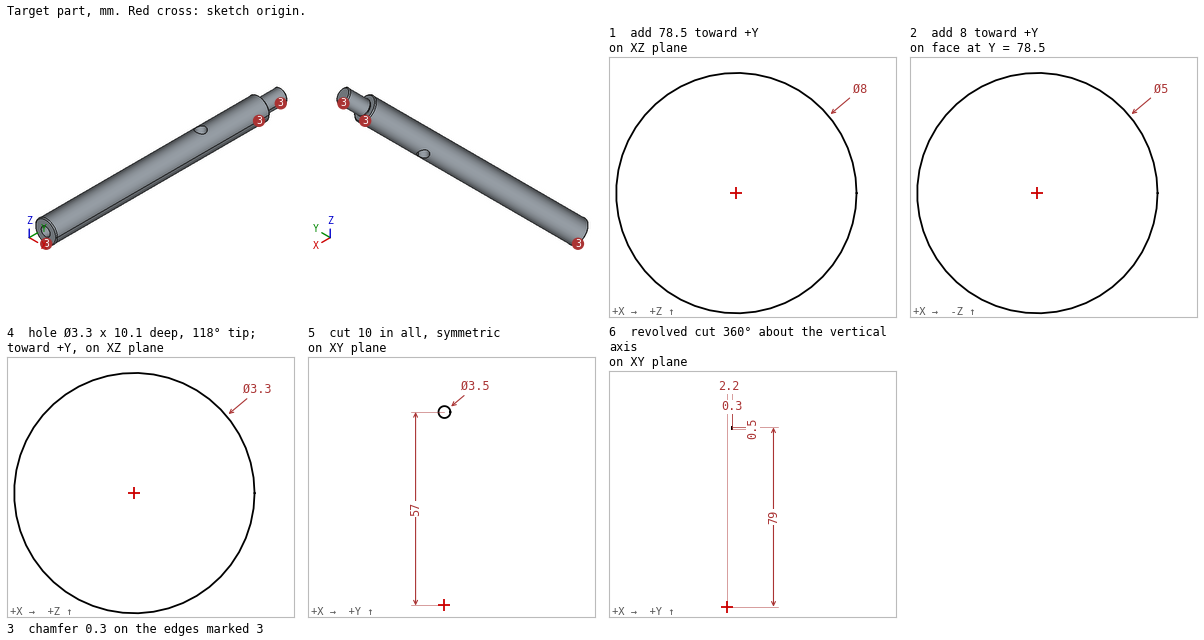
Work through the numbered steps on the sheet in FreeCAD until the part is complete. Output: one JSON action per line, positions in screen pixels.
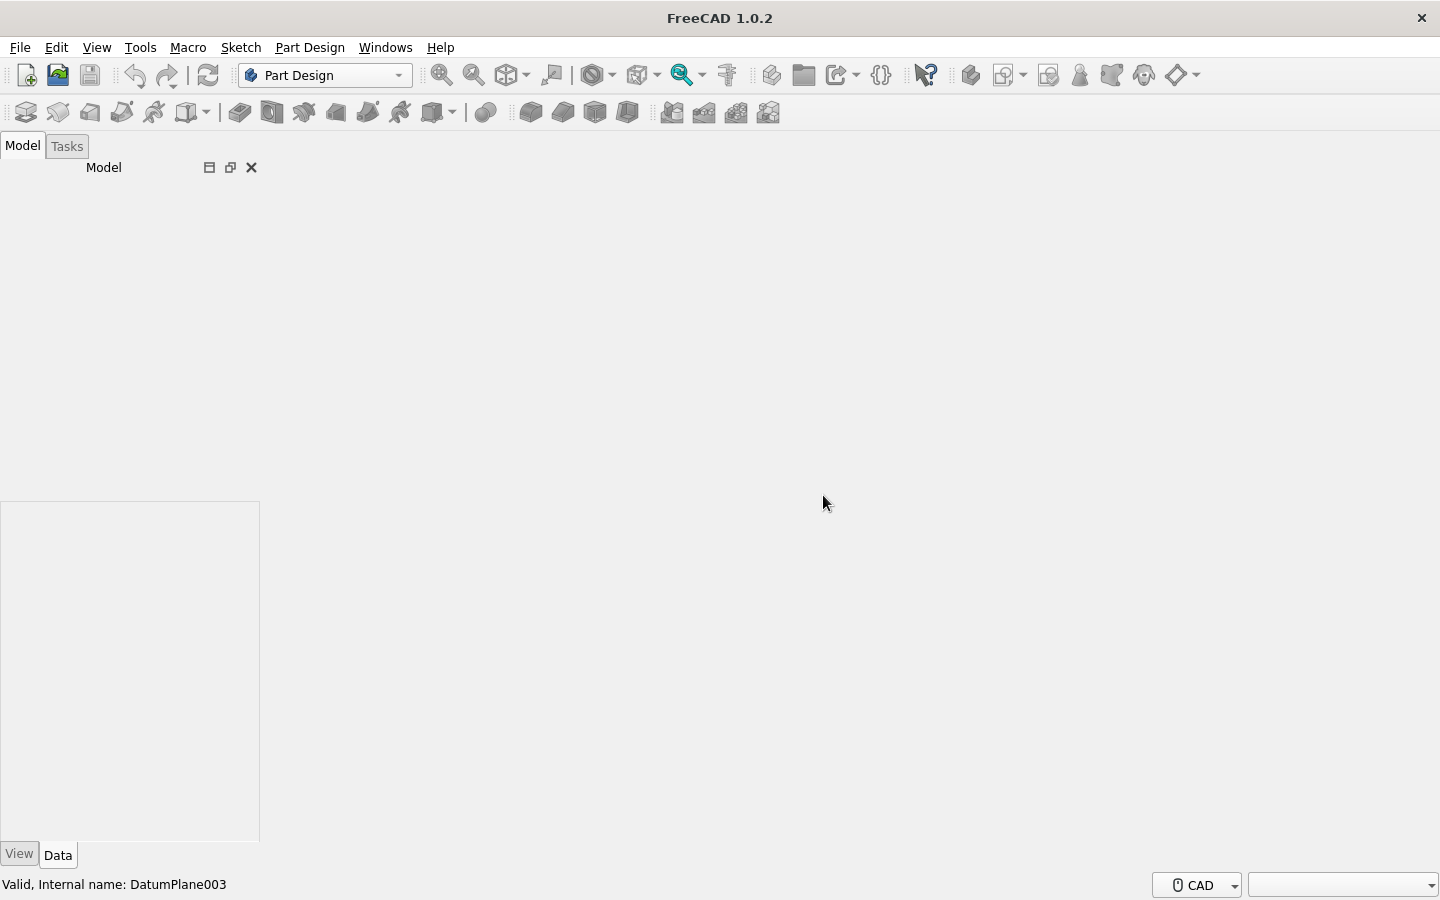
{"action": "left_click", "coordinate": [26, 76]}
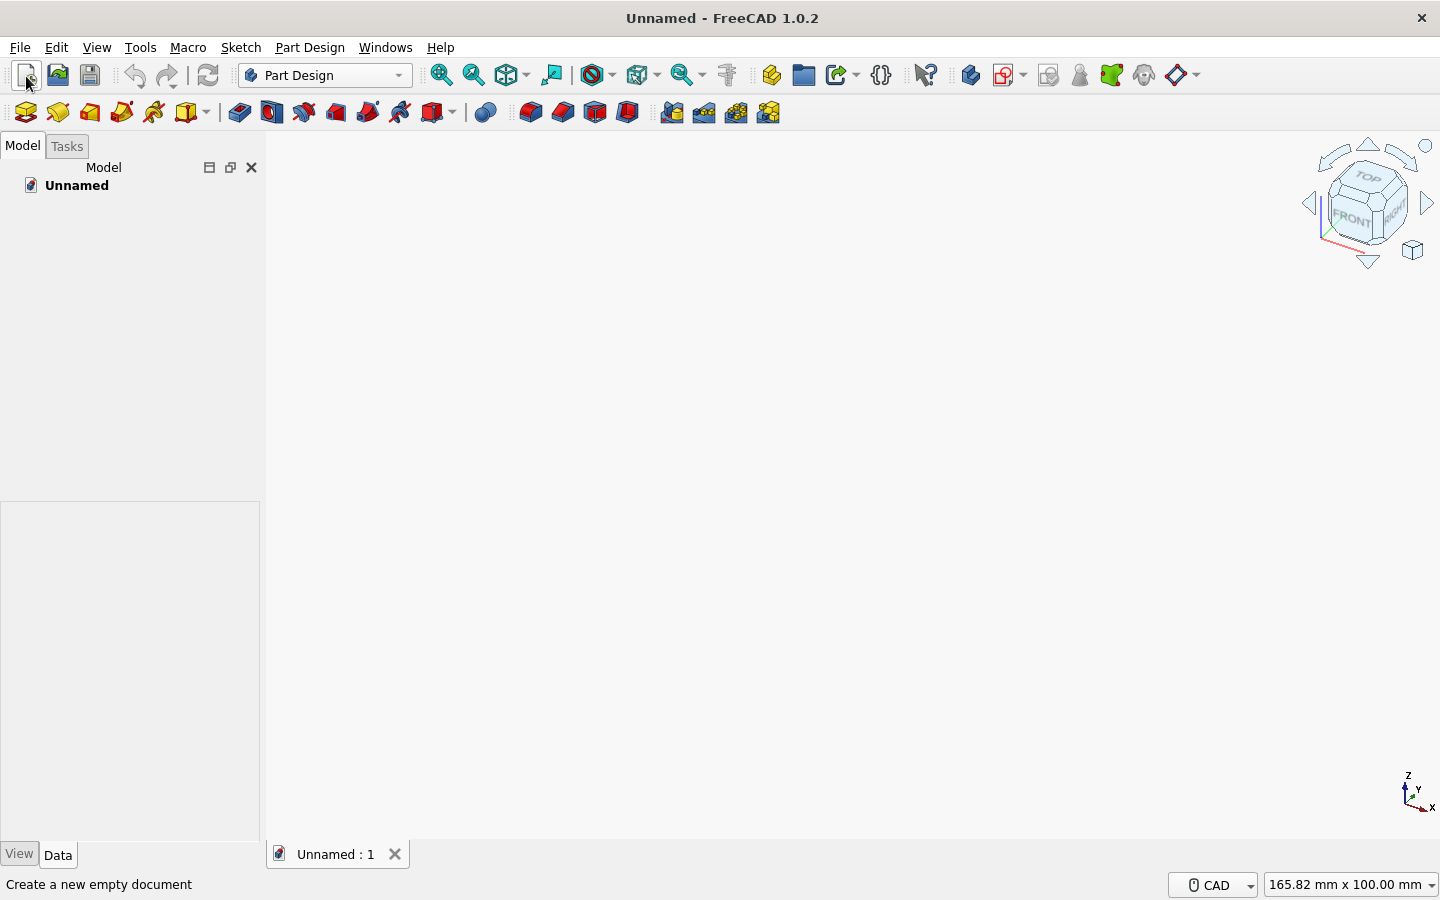
{"action": "left_click", "coordinate": [1004, 76]}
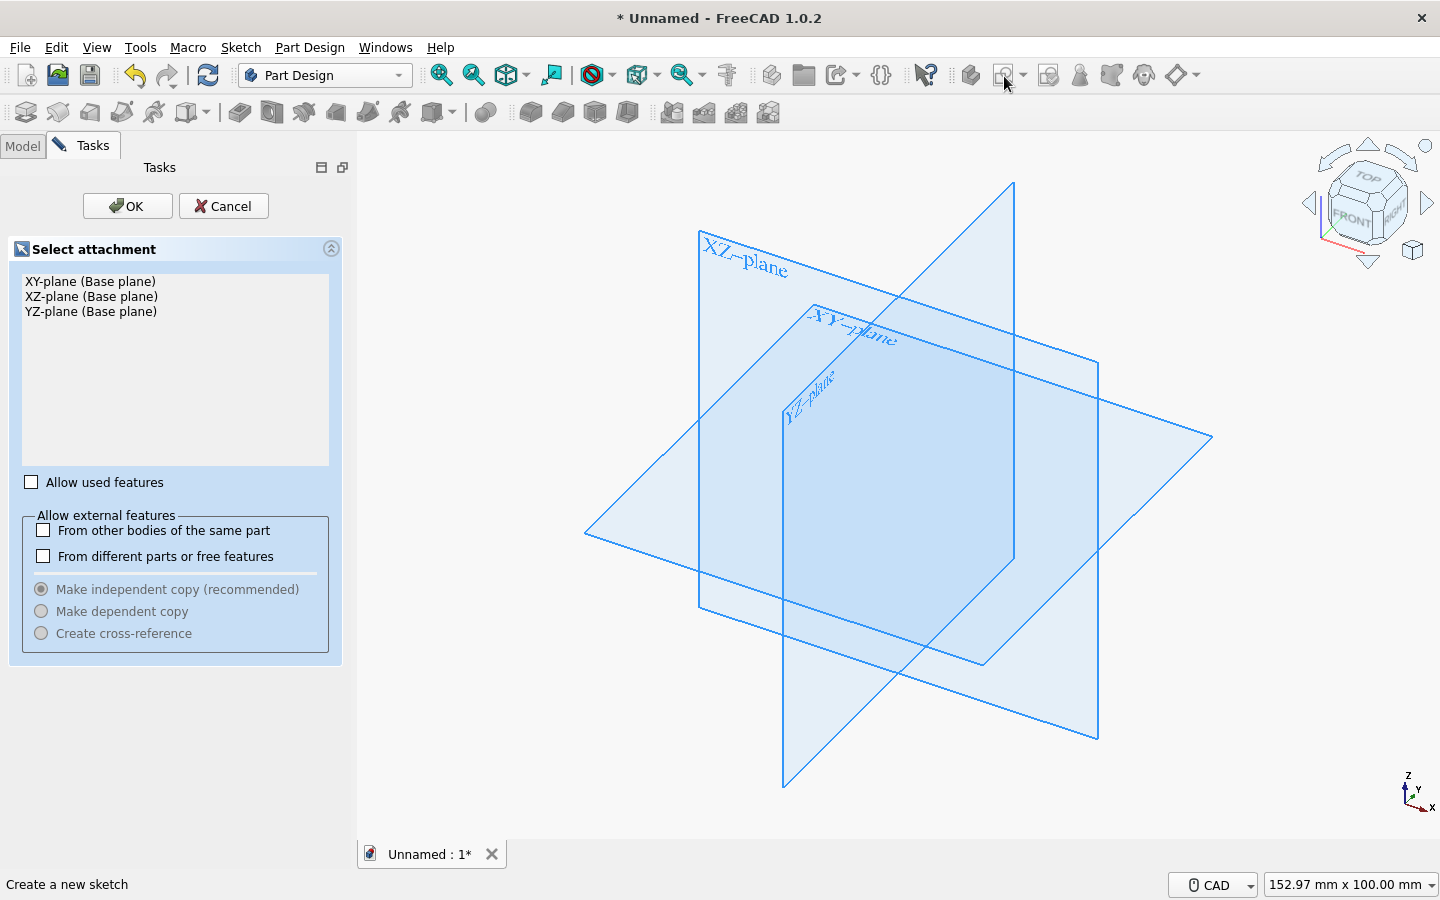
{"action": "left_click", "coordinate": [82, 296]}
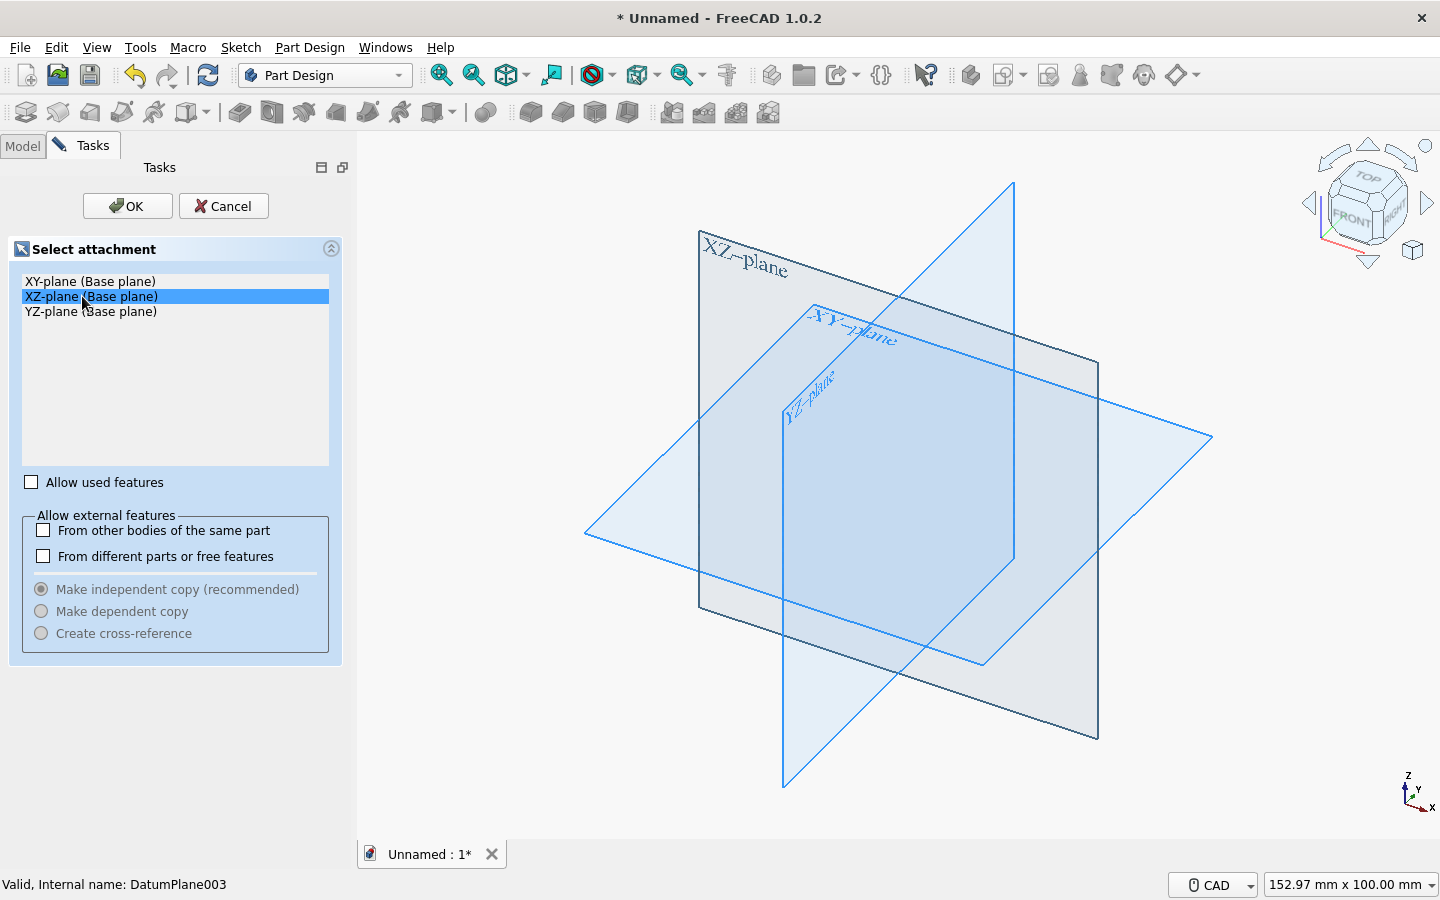
{"action": "left_click", "coordinate": [128, 206]}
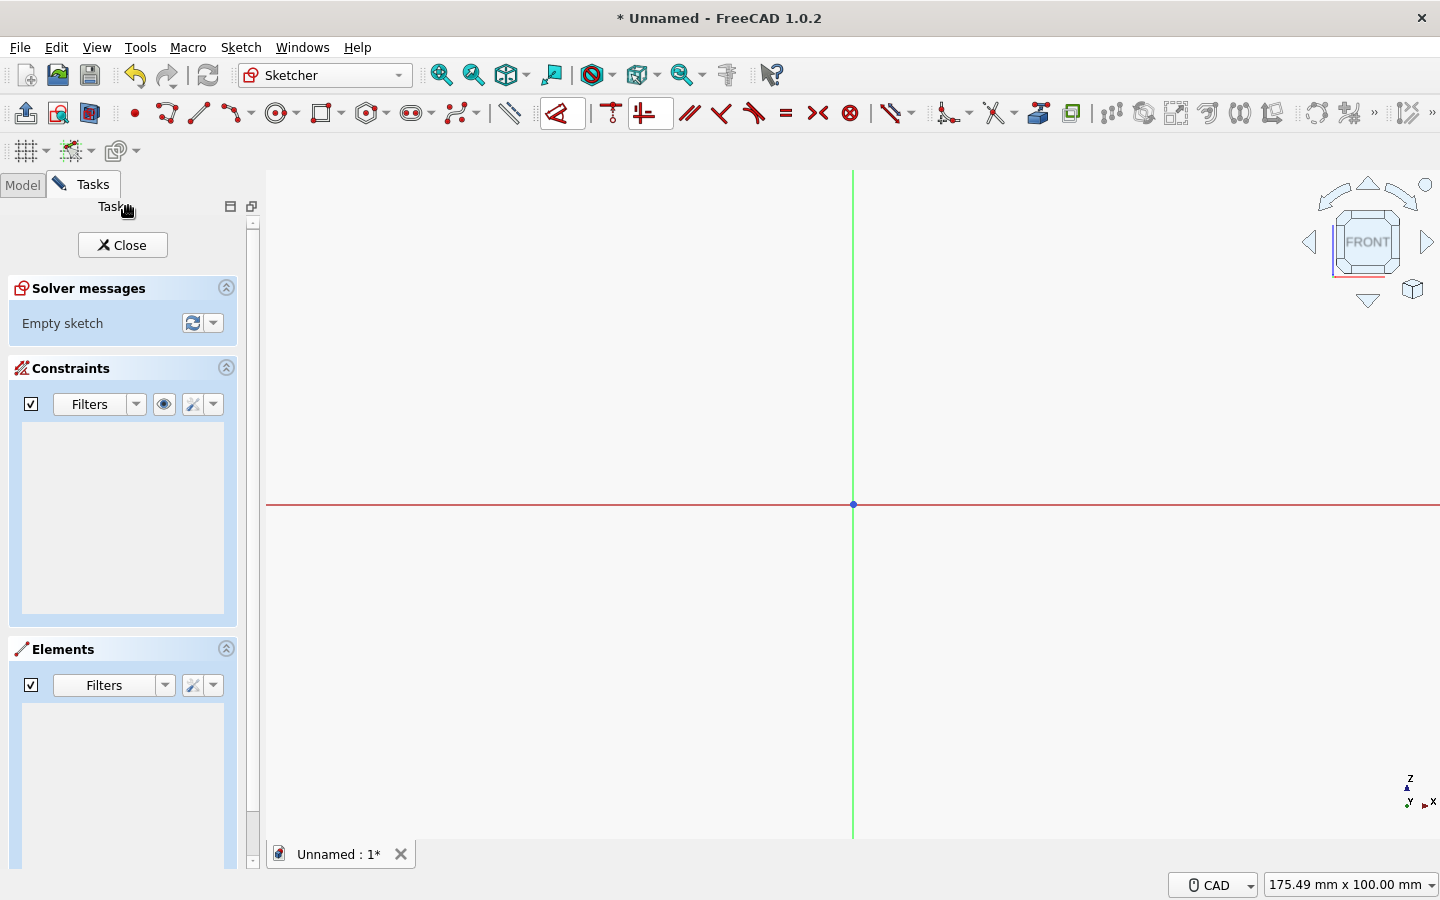
{"action": "scroll", "coordinate": [864, 504], "scroll_direction": "up", "scroll_amount": 10}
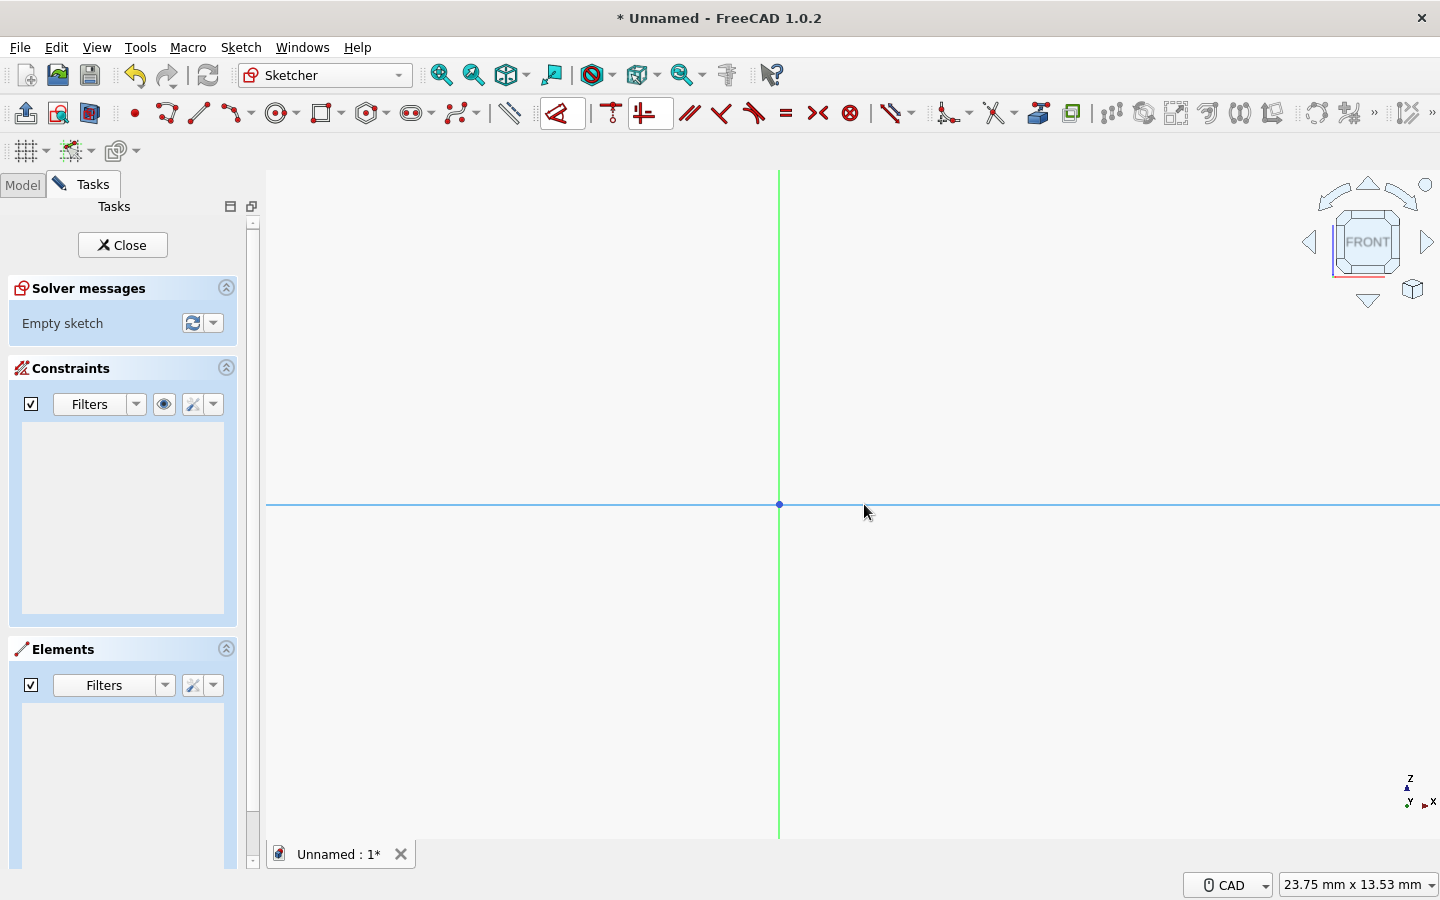
{"action": "key", "text": "g c"}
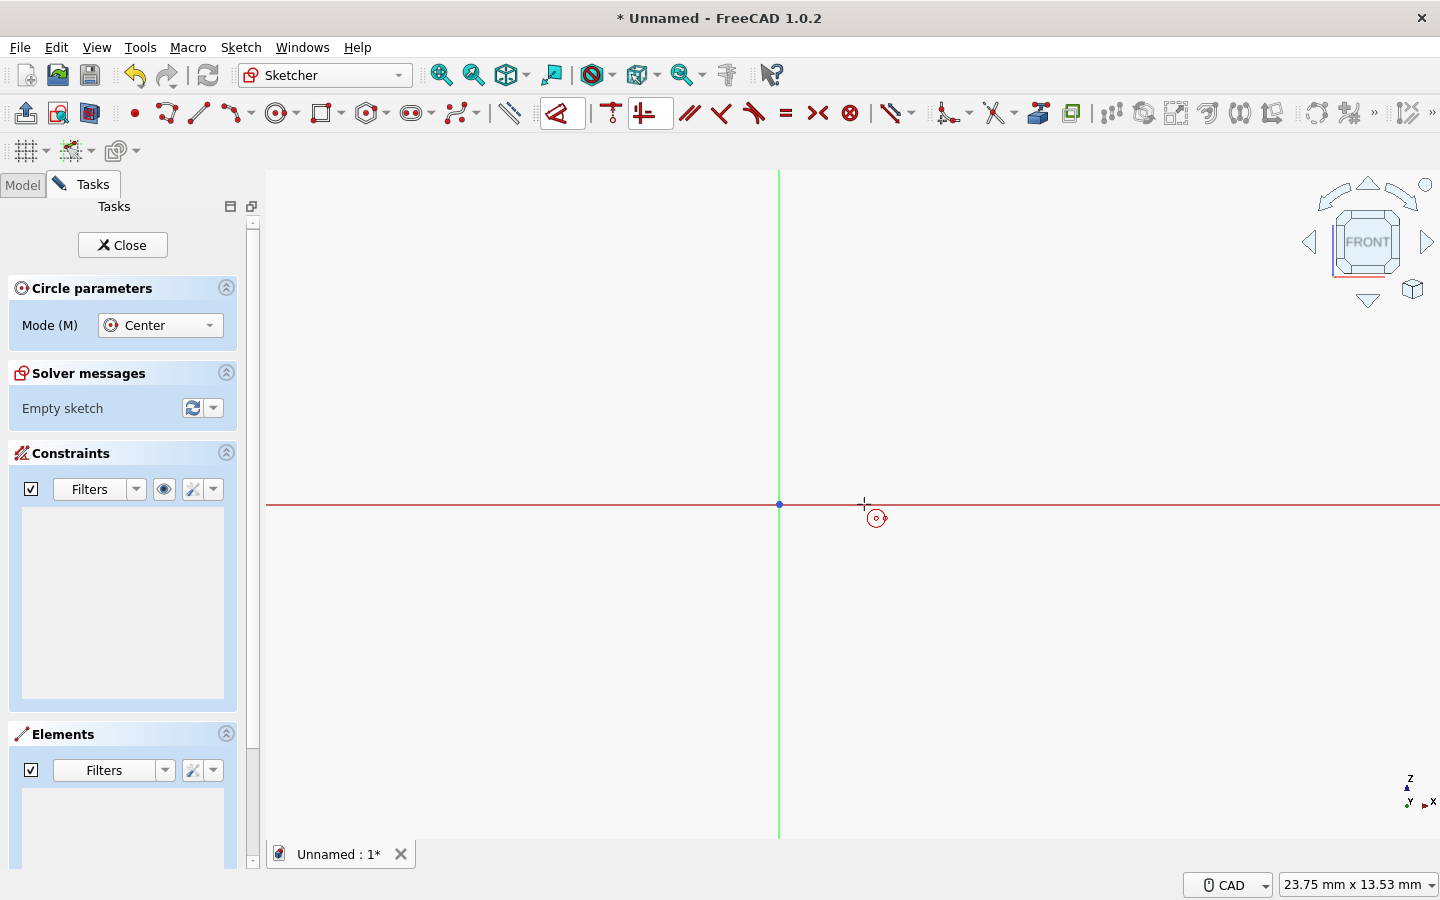
{"action": "left_click", "coordinate": [779, 504]}
{"action": "left_click", "coordinate": [919, 365]}
{"action": "key", "text": "Escape"}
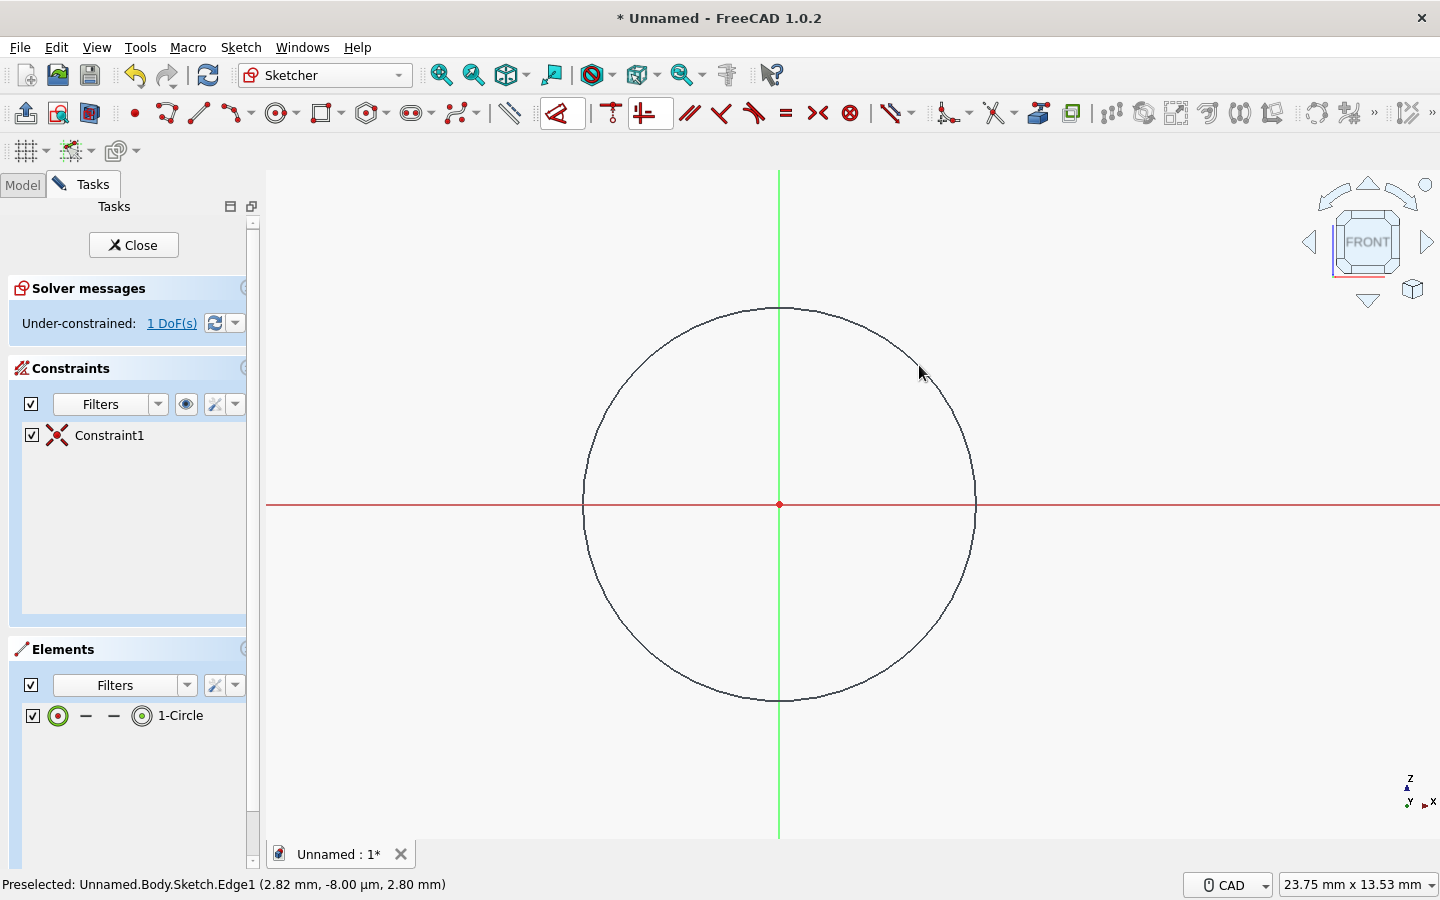
{"action": "key", "text": "d"}